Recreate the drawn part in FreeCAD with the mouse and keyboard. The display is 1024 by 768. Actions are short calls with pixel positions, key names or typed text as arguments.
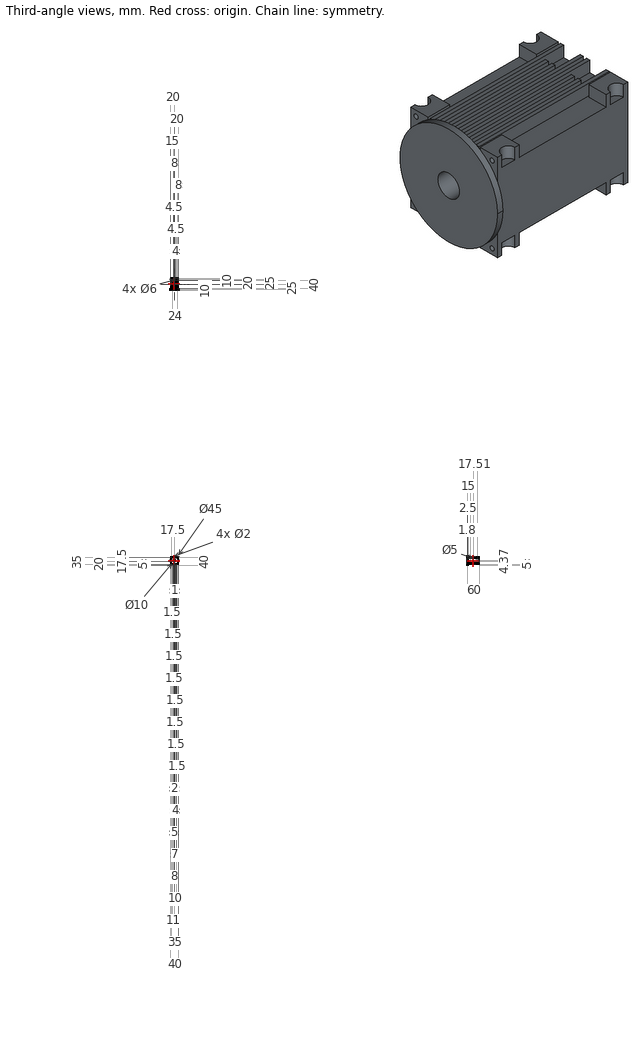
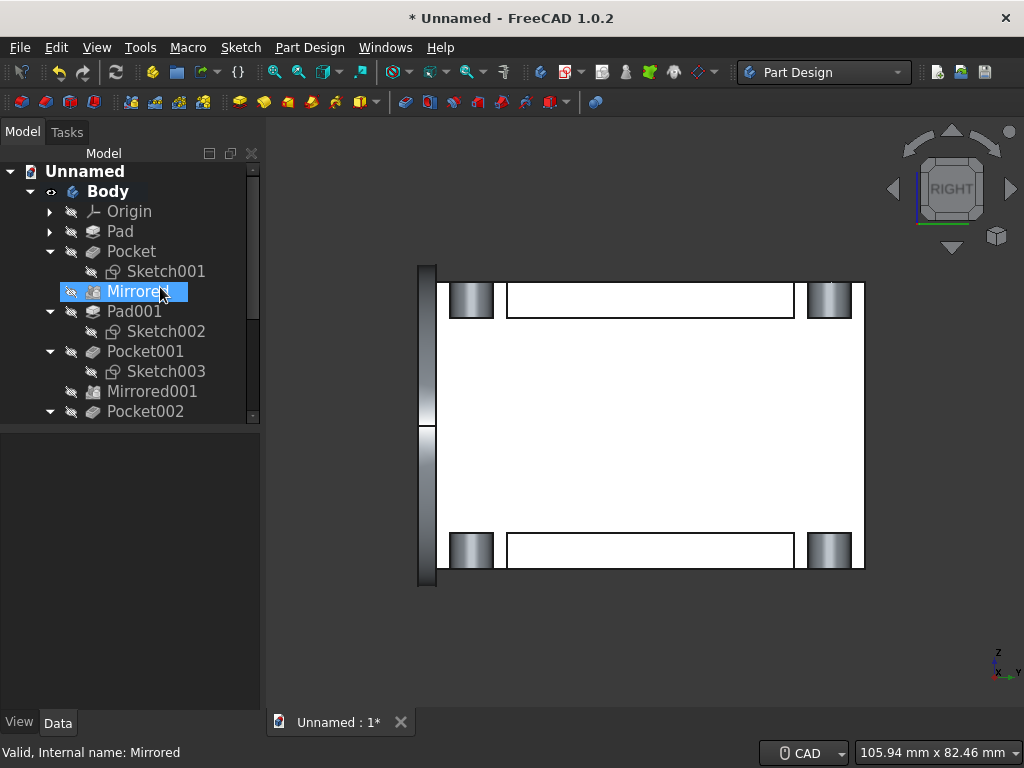
click(50, 212)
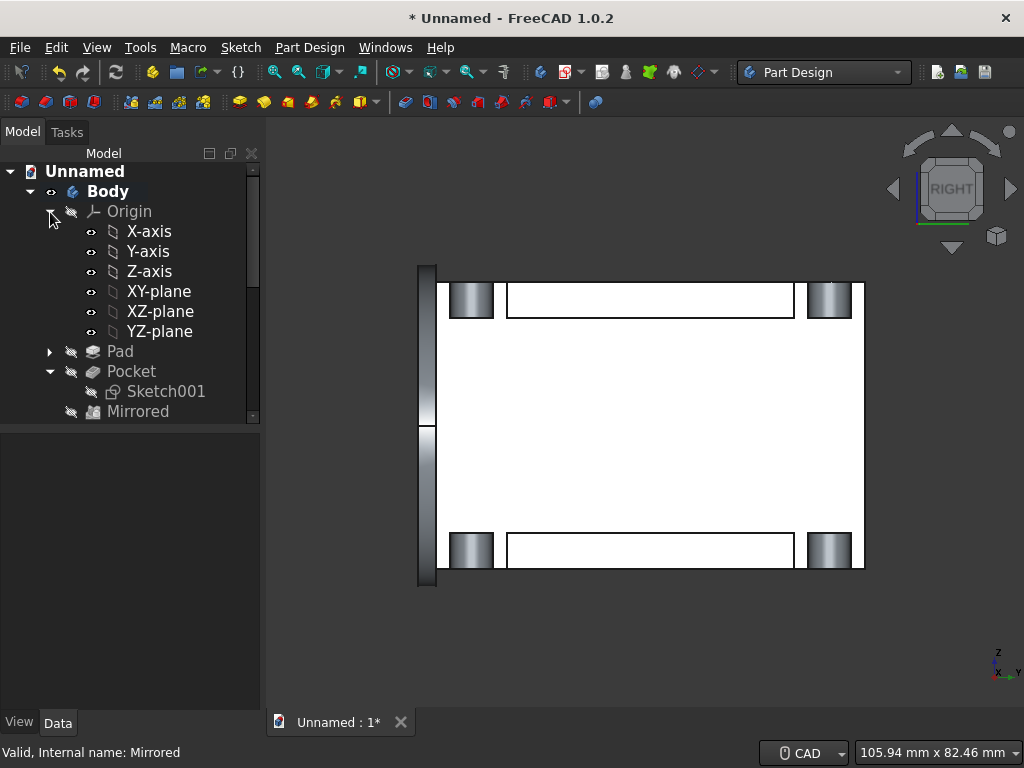
click(136, 312)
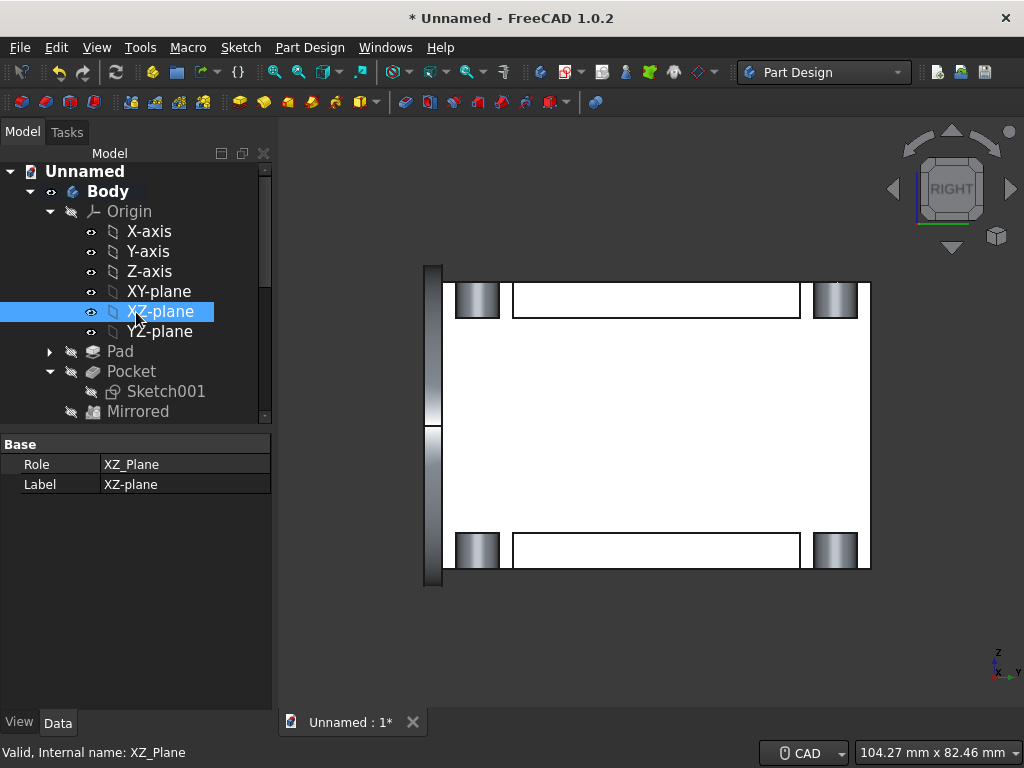
click(698, 72)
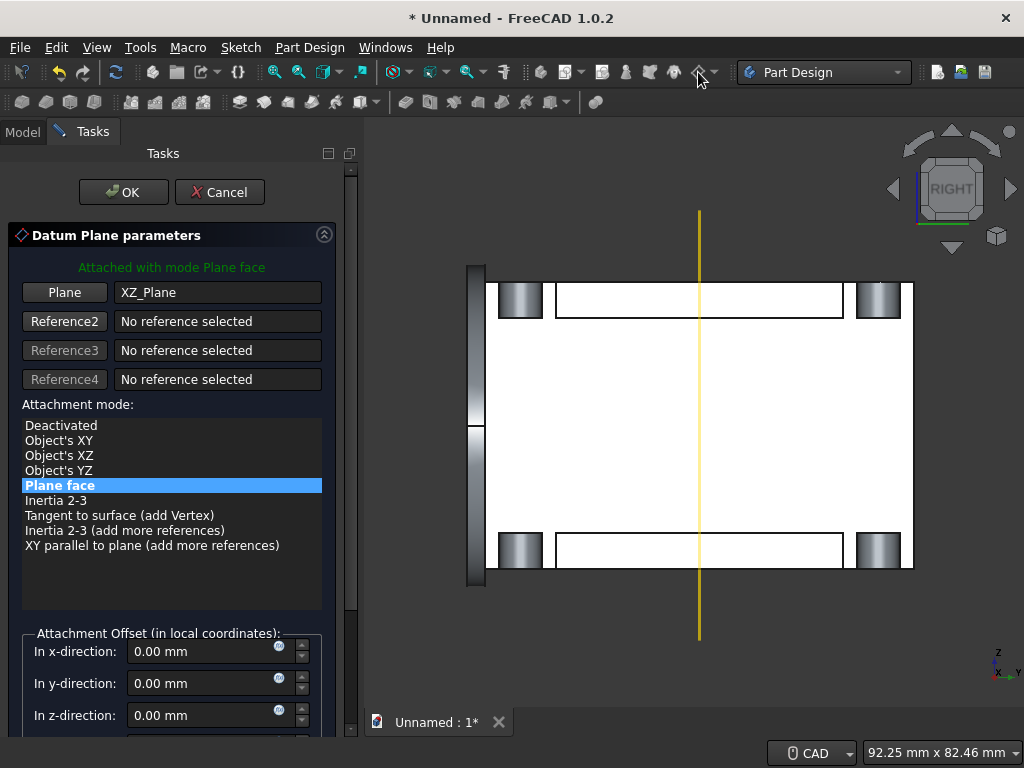
triple_click(210, 715)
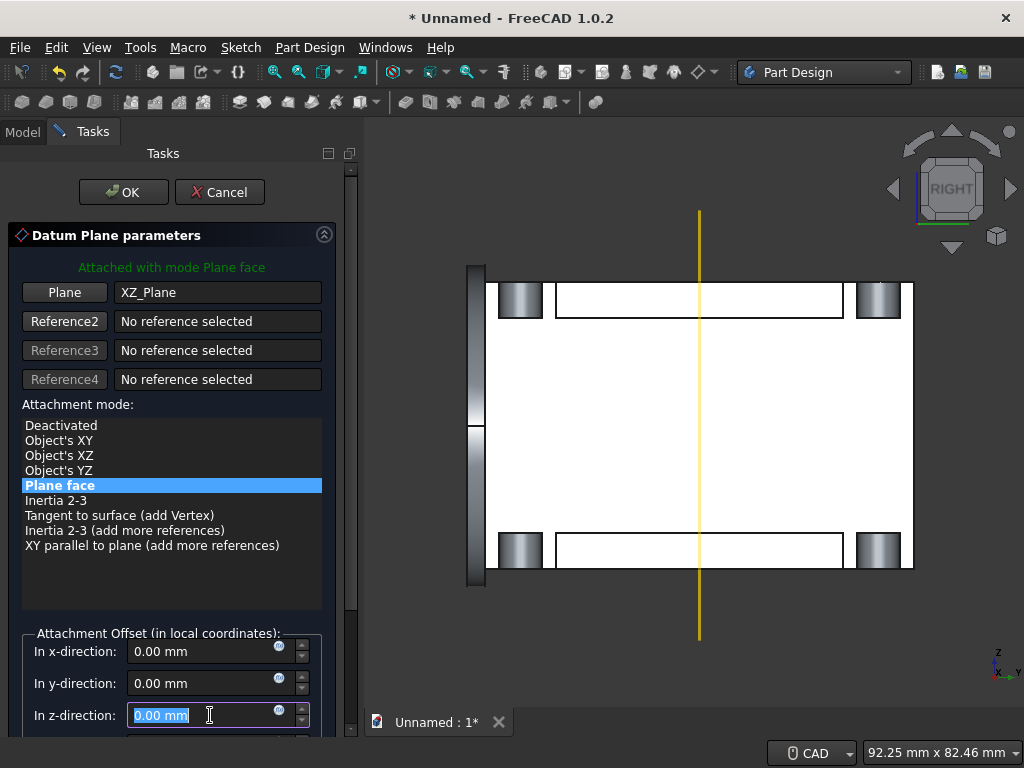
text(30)
key(Tab)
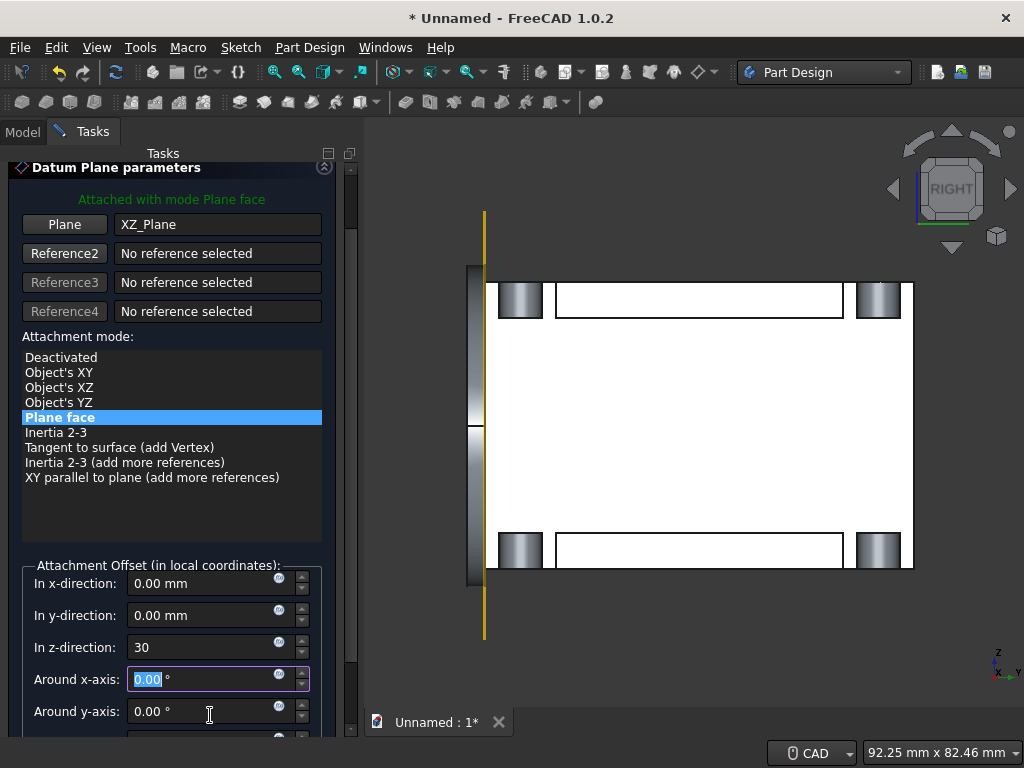
scroll(351, 450, up, 2)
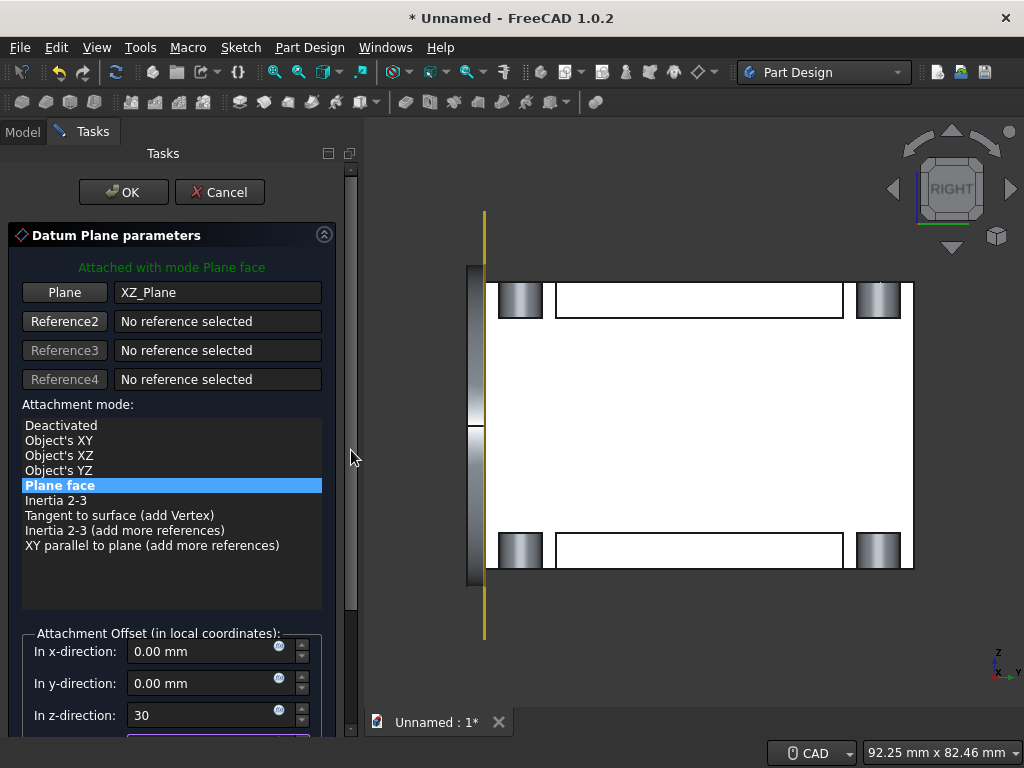
click(124, 192)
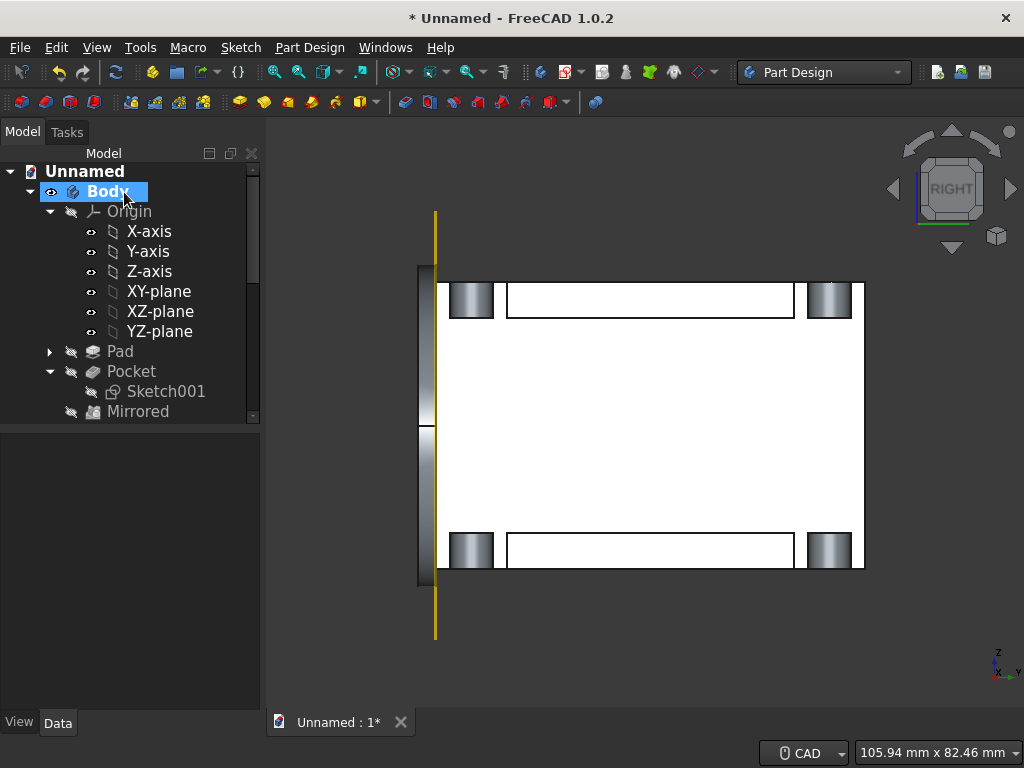
scroll(100, 287, down, 3)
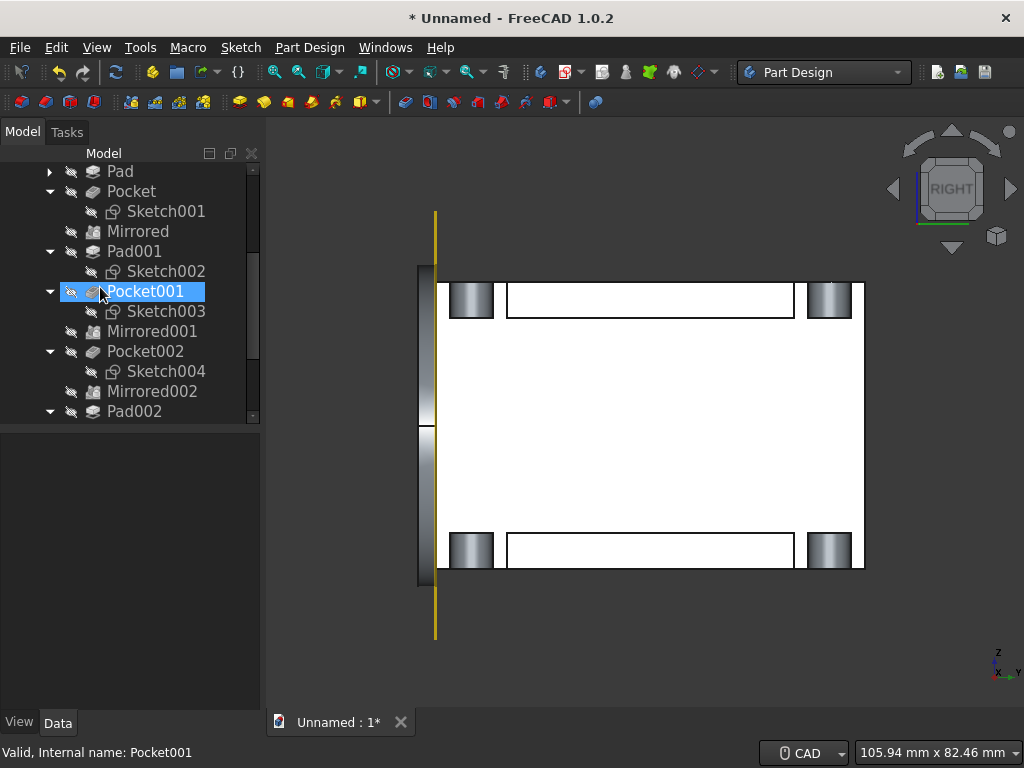
scroll(140, 287, up, 15)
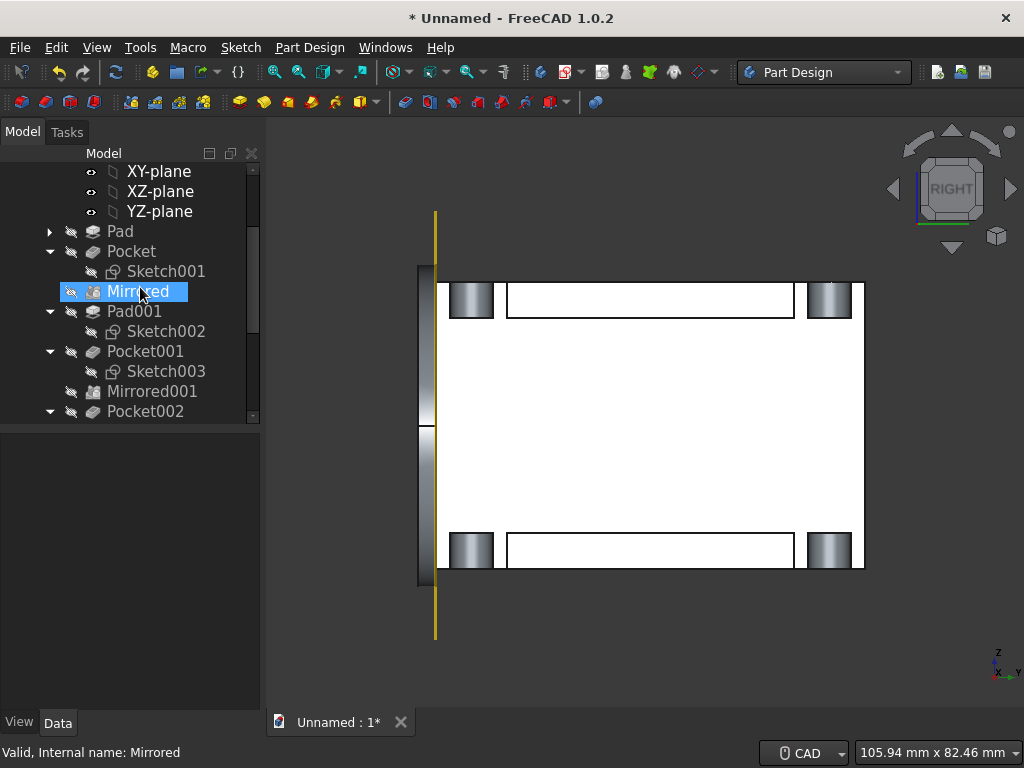
scroll(100, 287, down, 6)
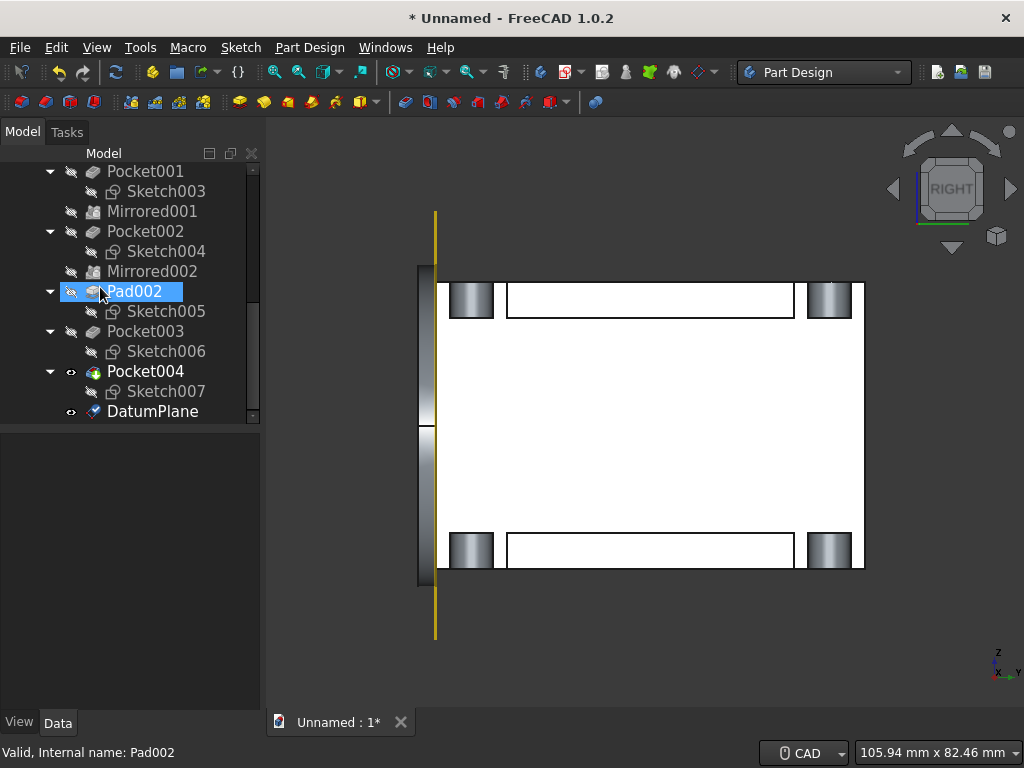
click(116, 412)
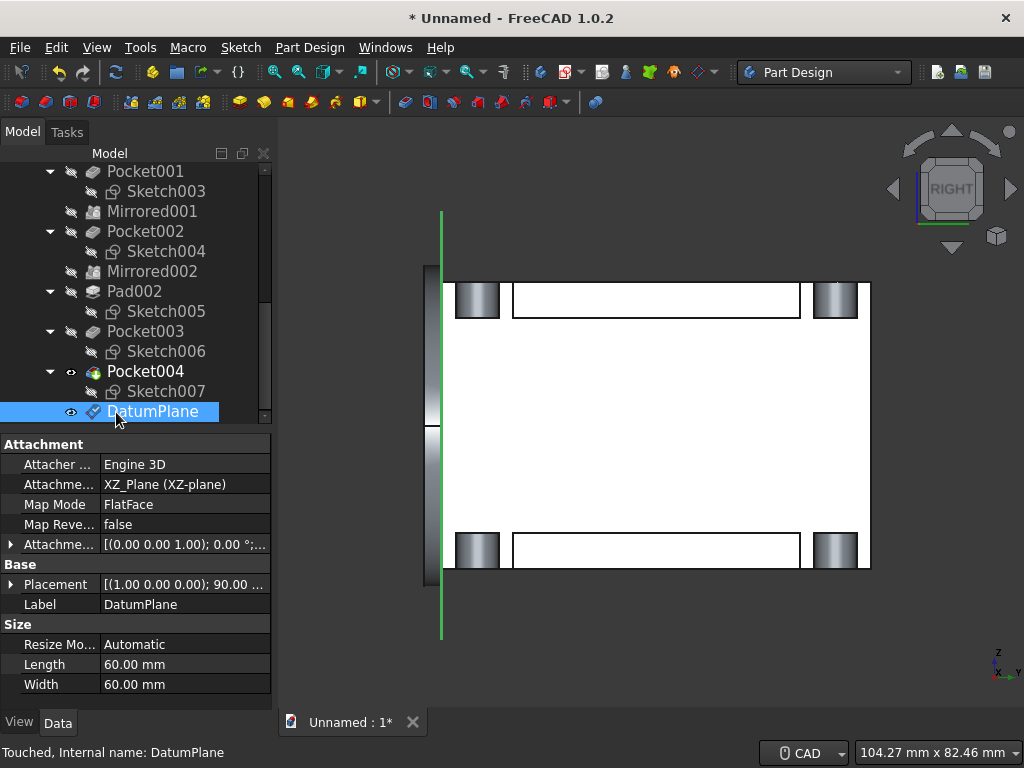
click(566, 72)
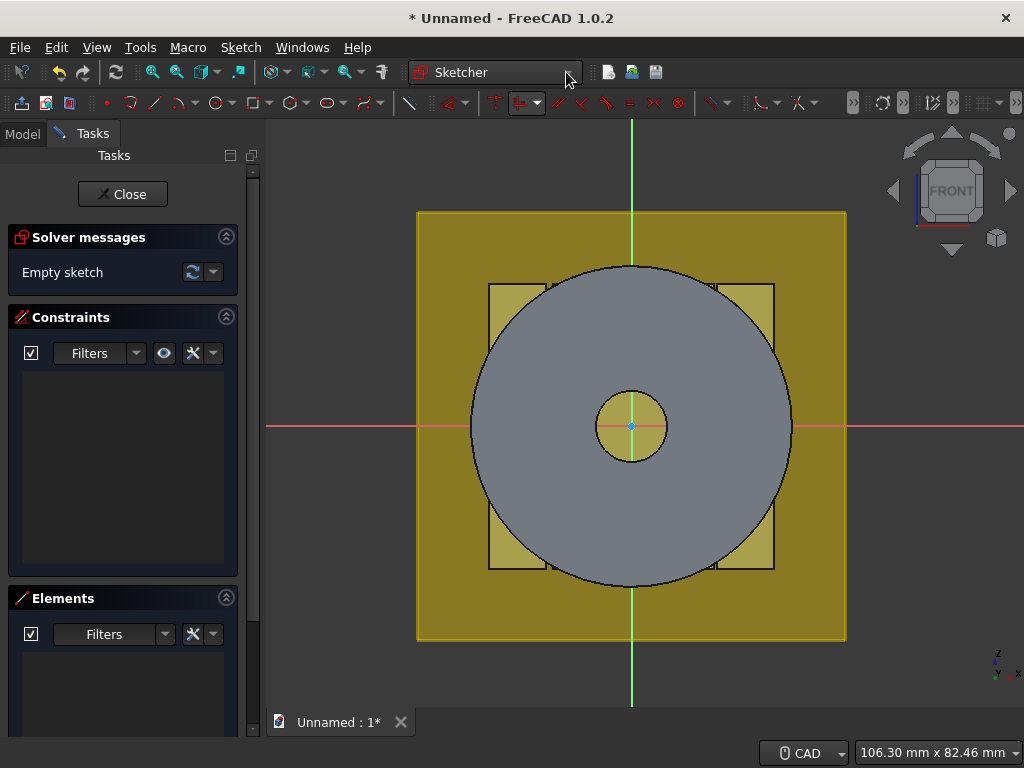
click(70, 104)